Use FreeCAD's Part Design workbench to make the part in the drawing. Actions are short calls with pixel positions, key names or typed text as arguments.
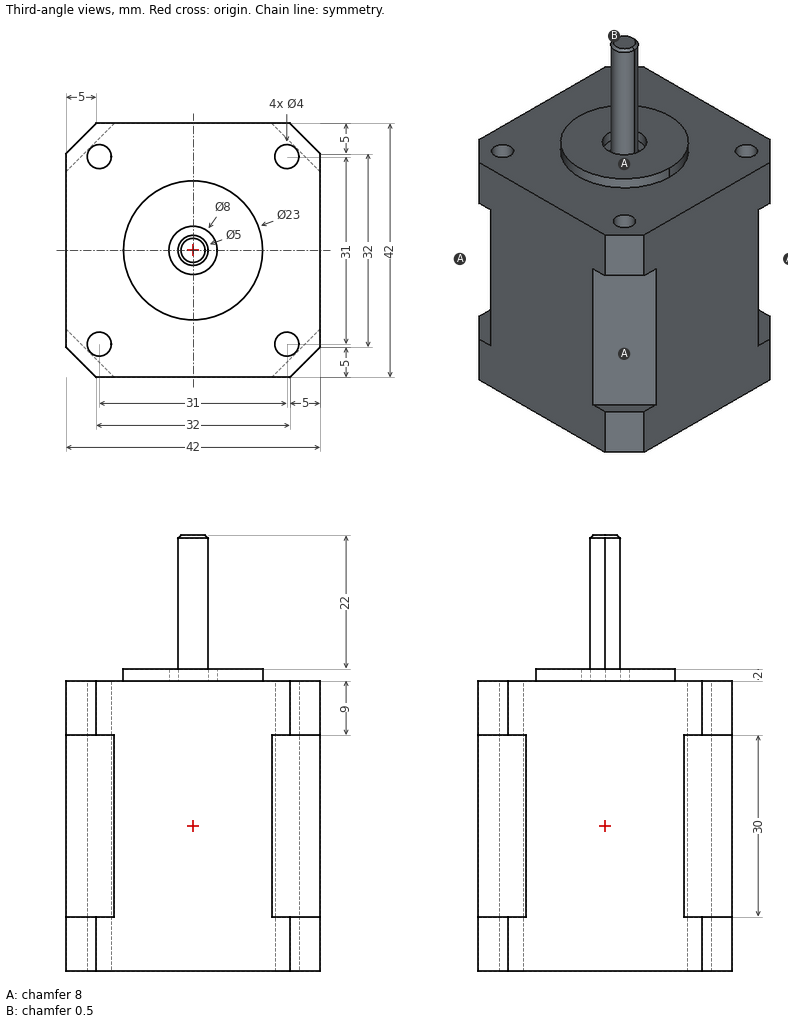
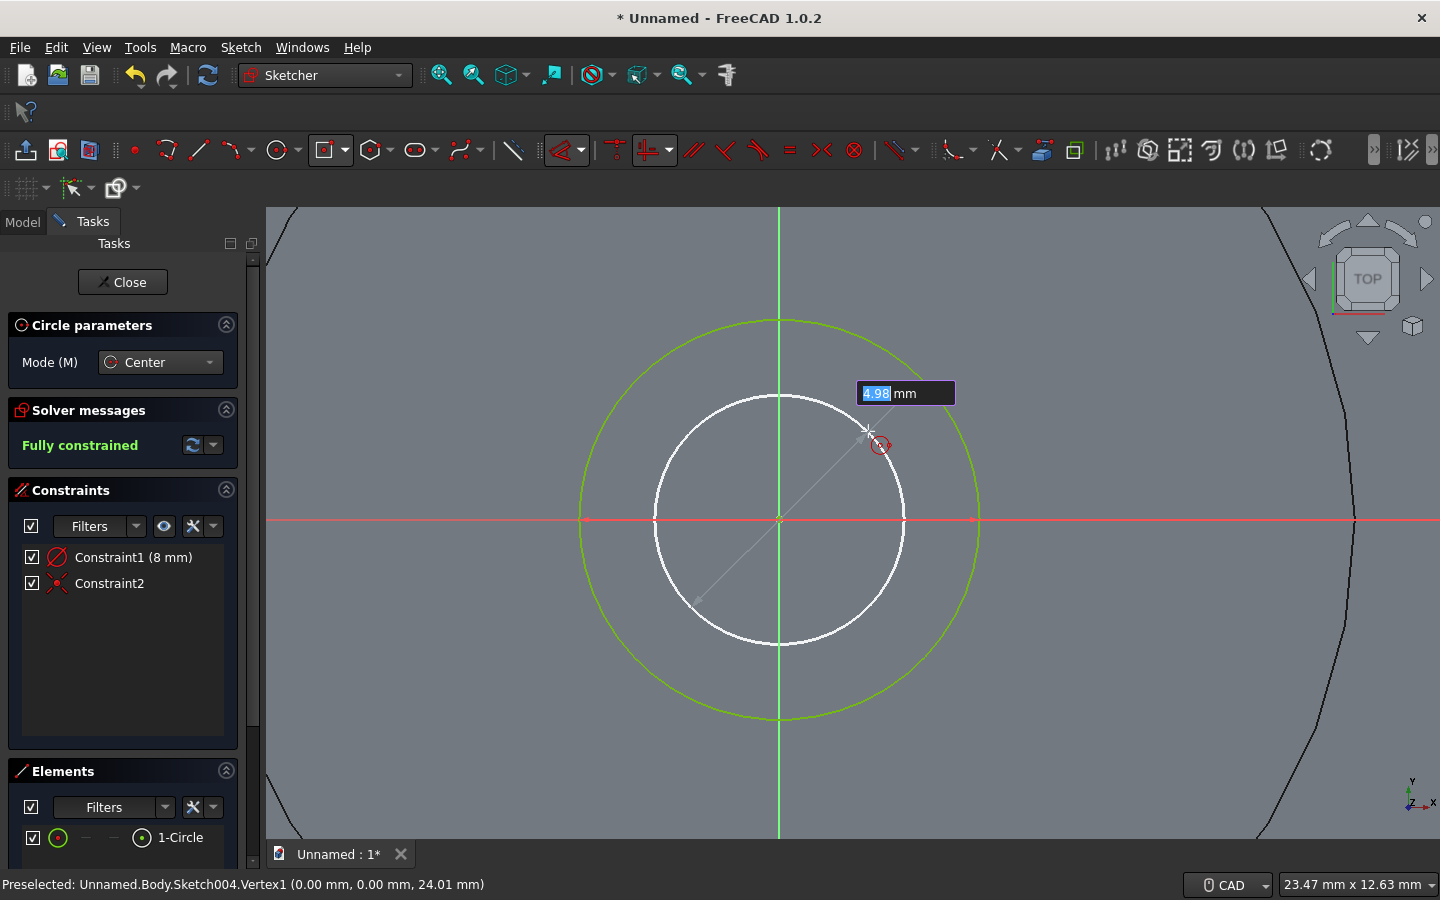
text(5)
key(Return)
key(Escape)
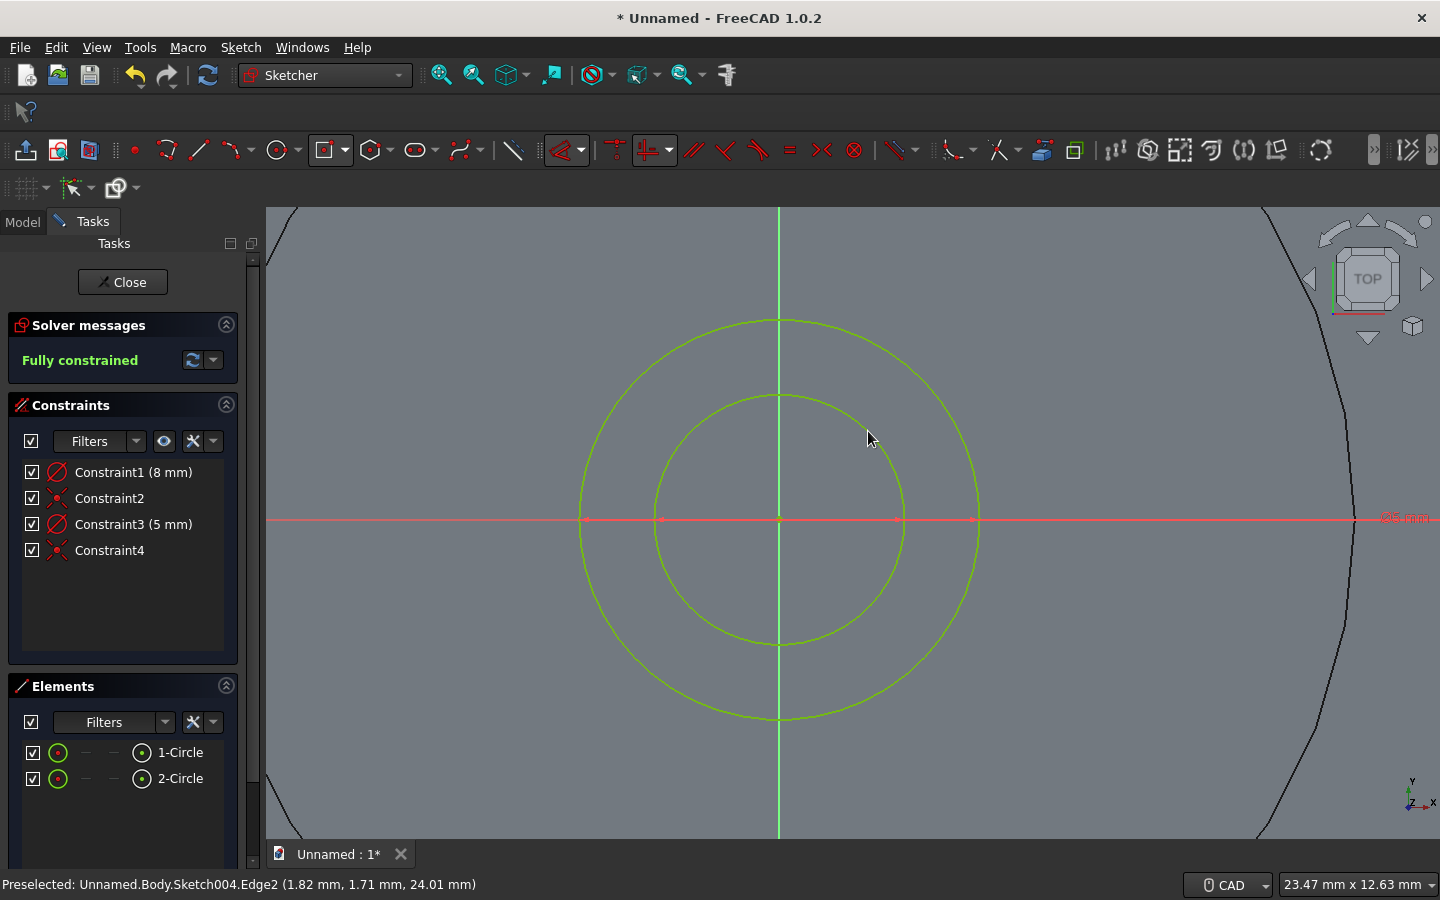
click(123, 282)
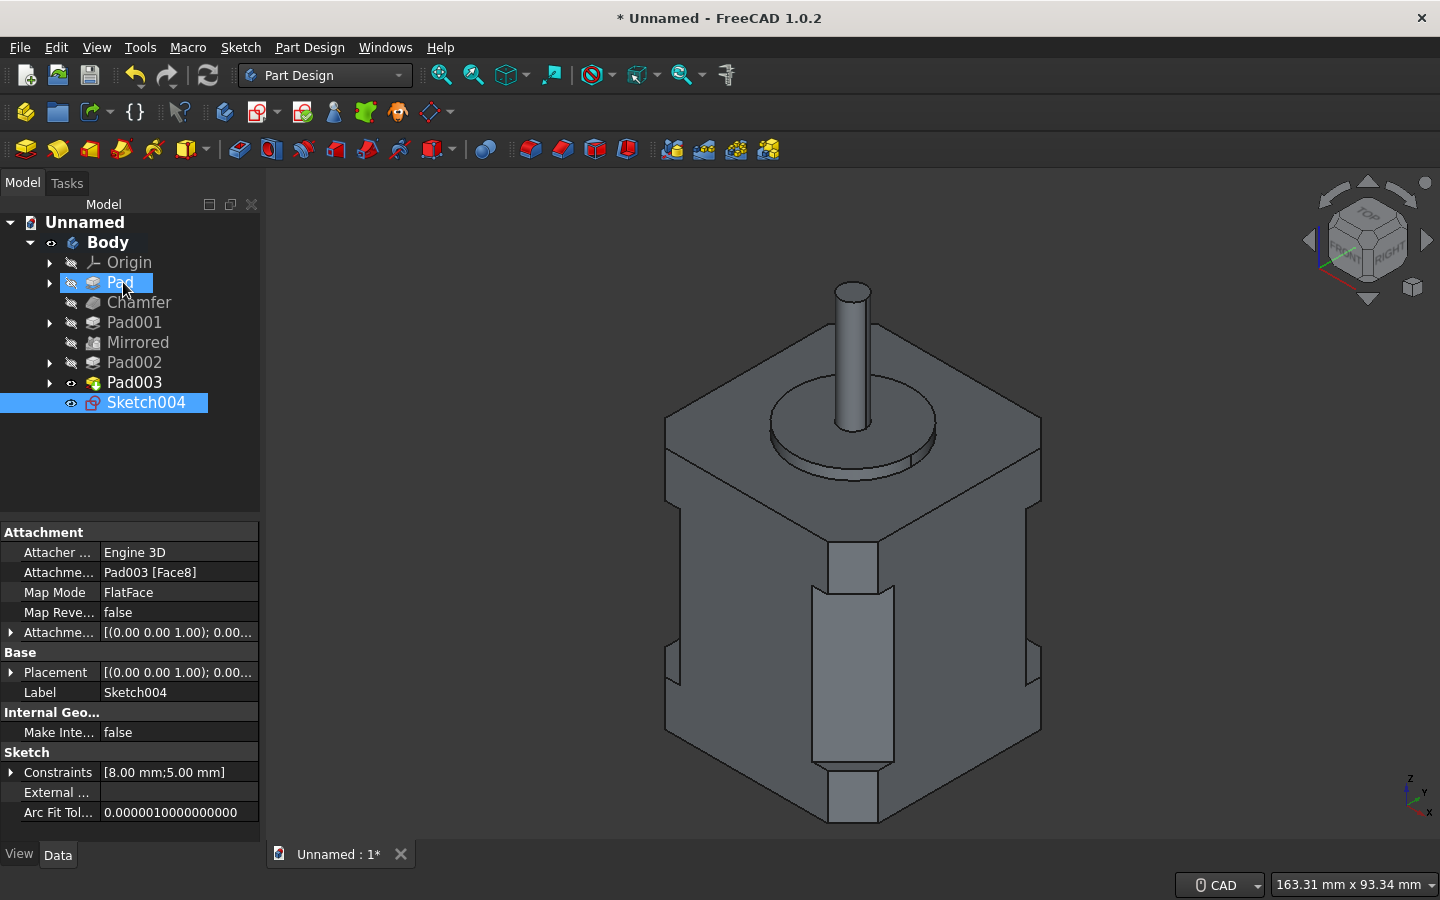
click(240, 150)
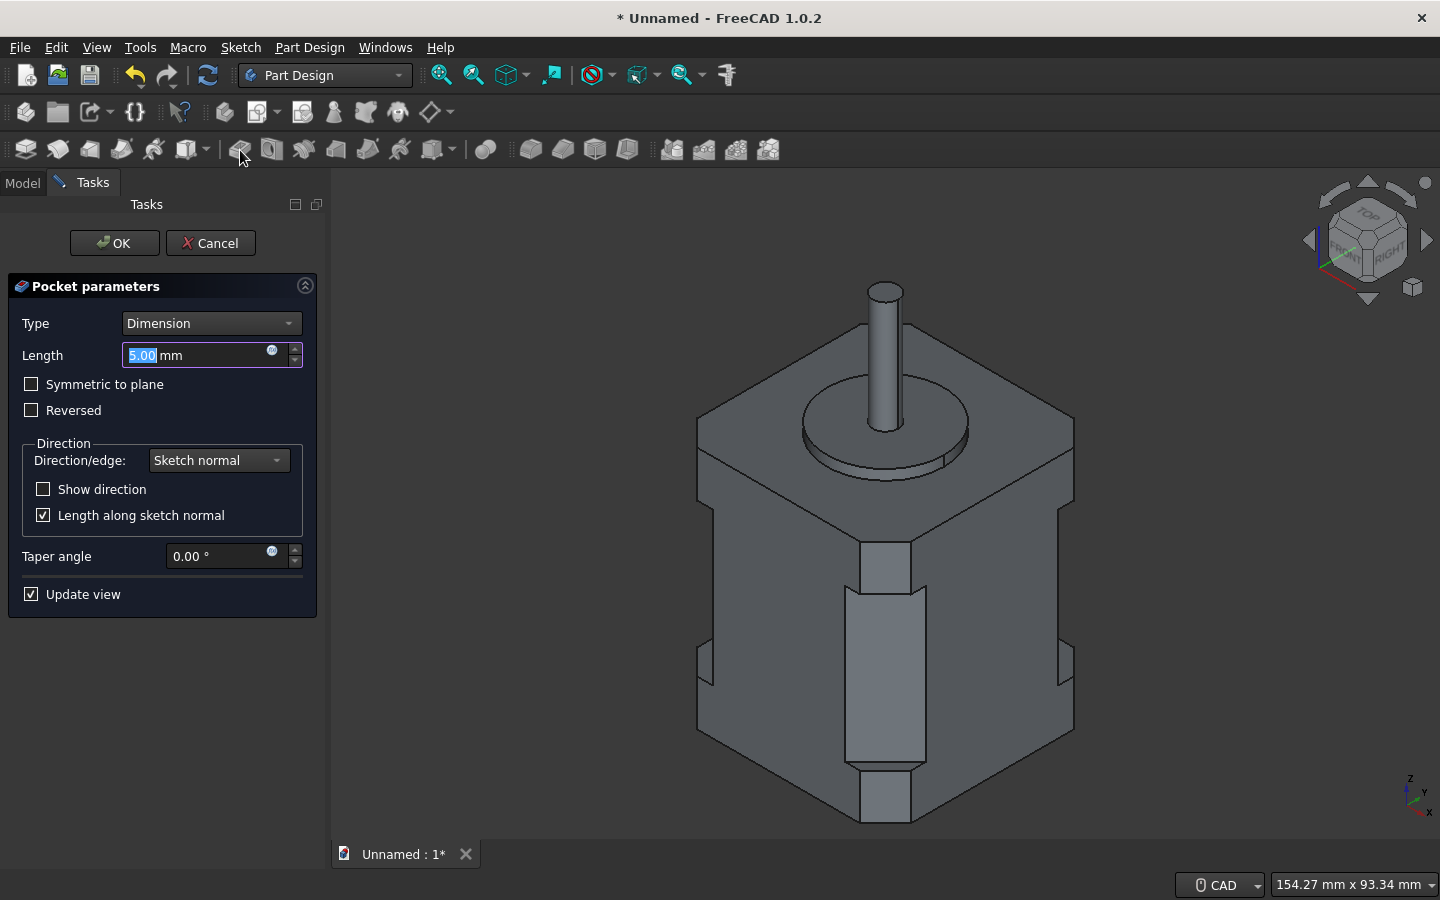
text(2)
key(Tab)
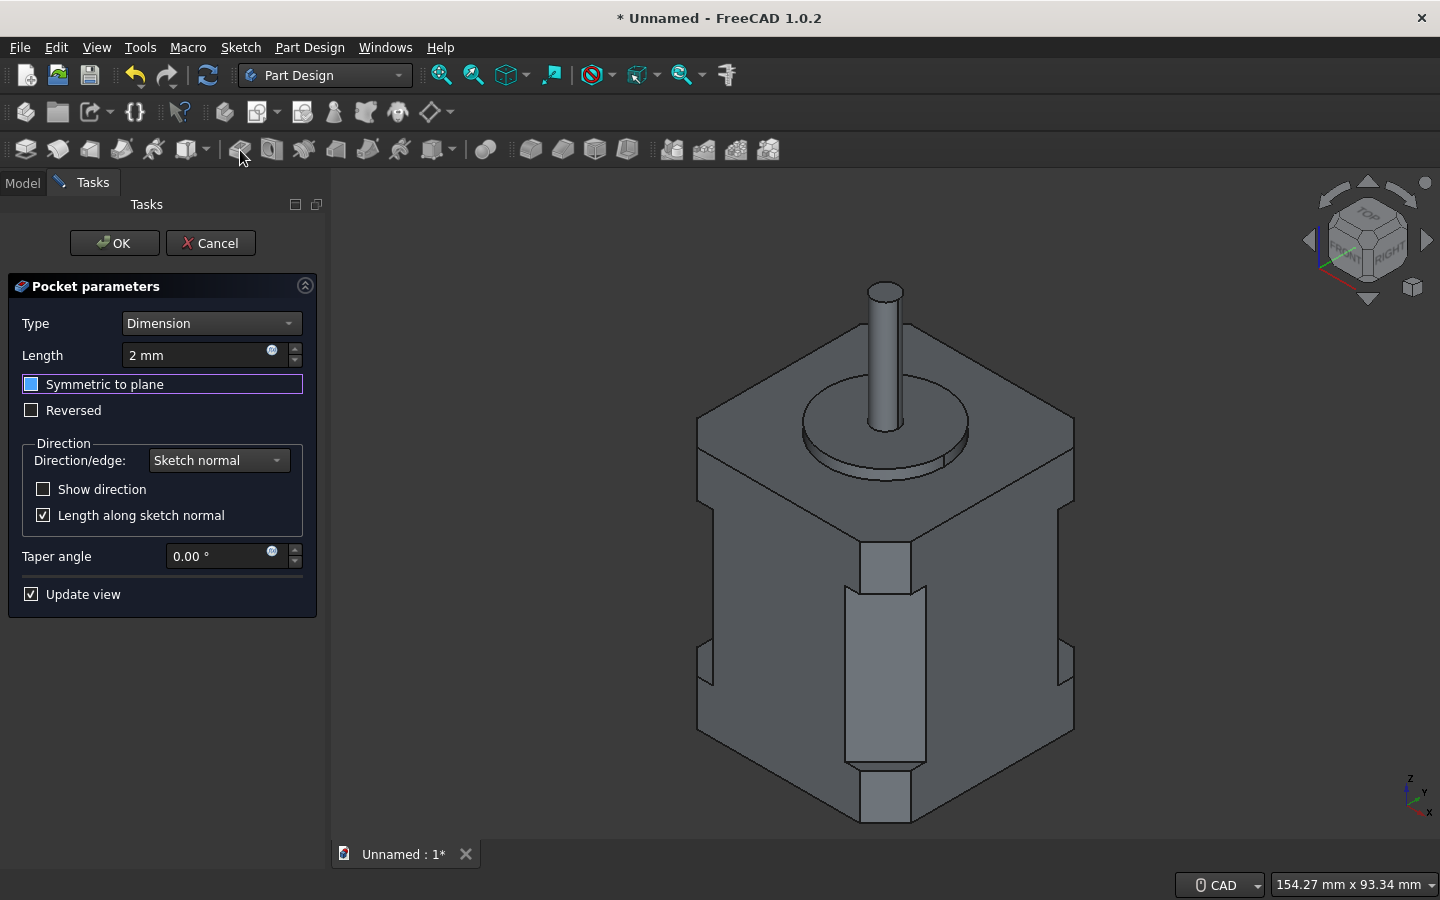
click(30, 410)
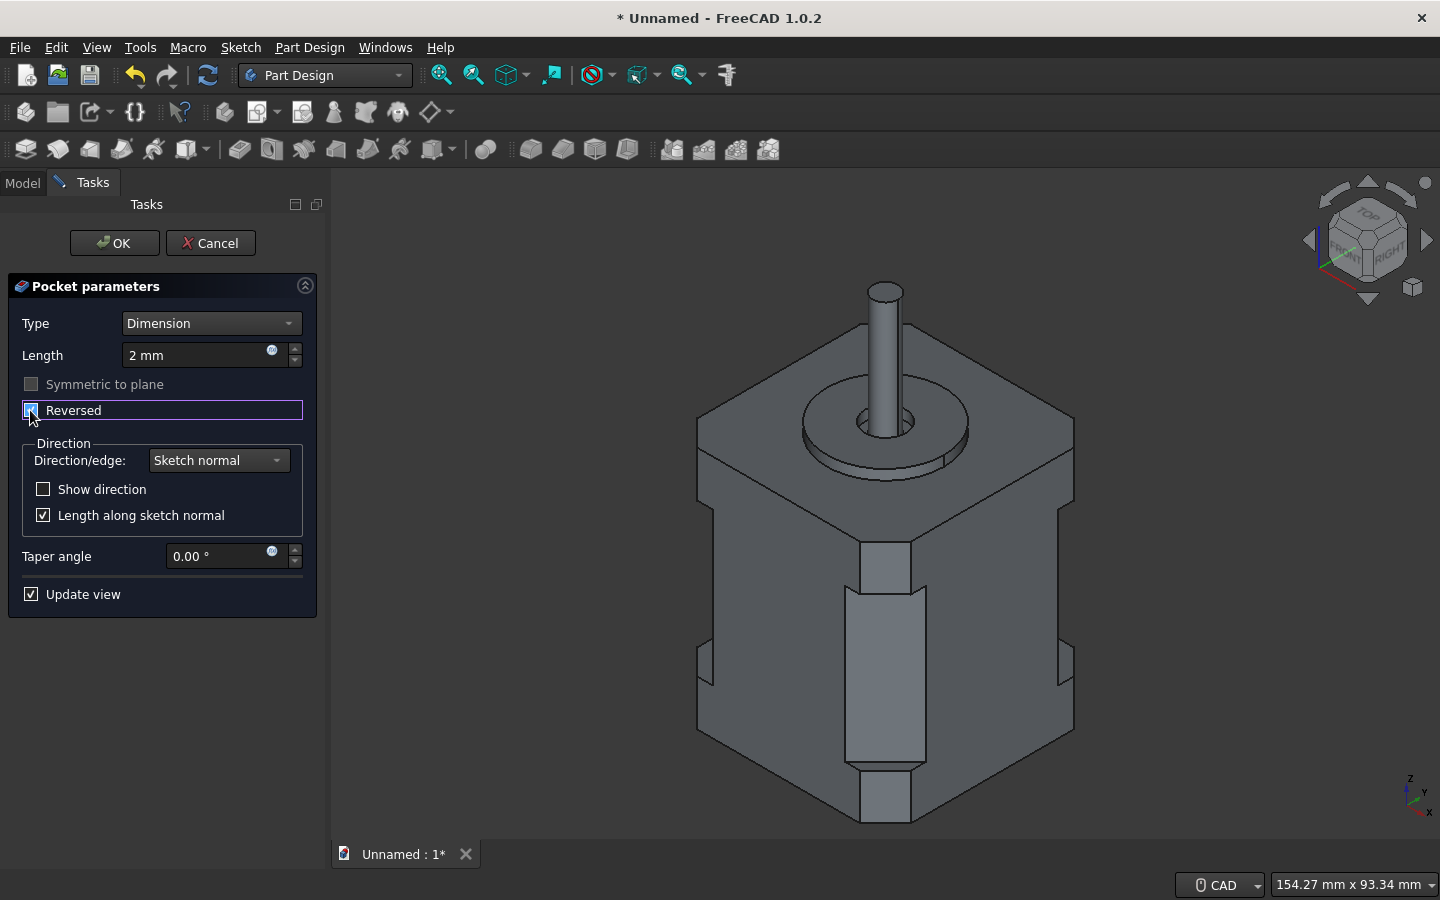
click(115, 243)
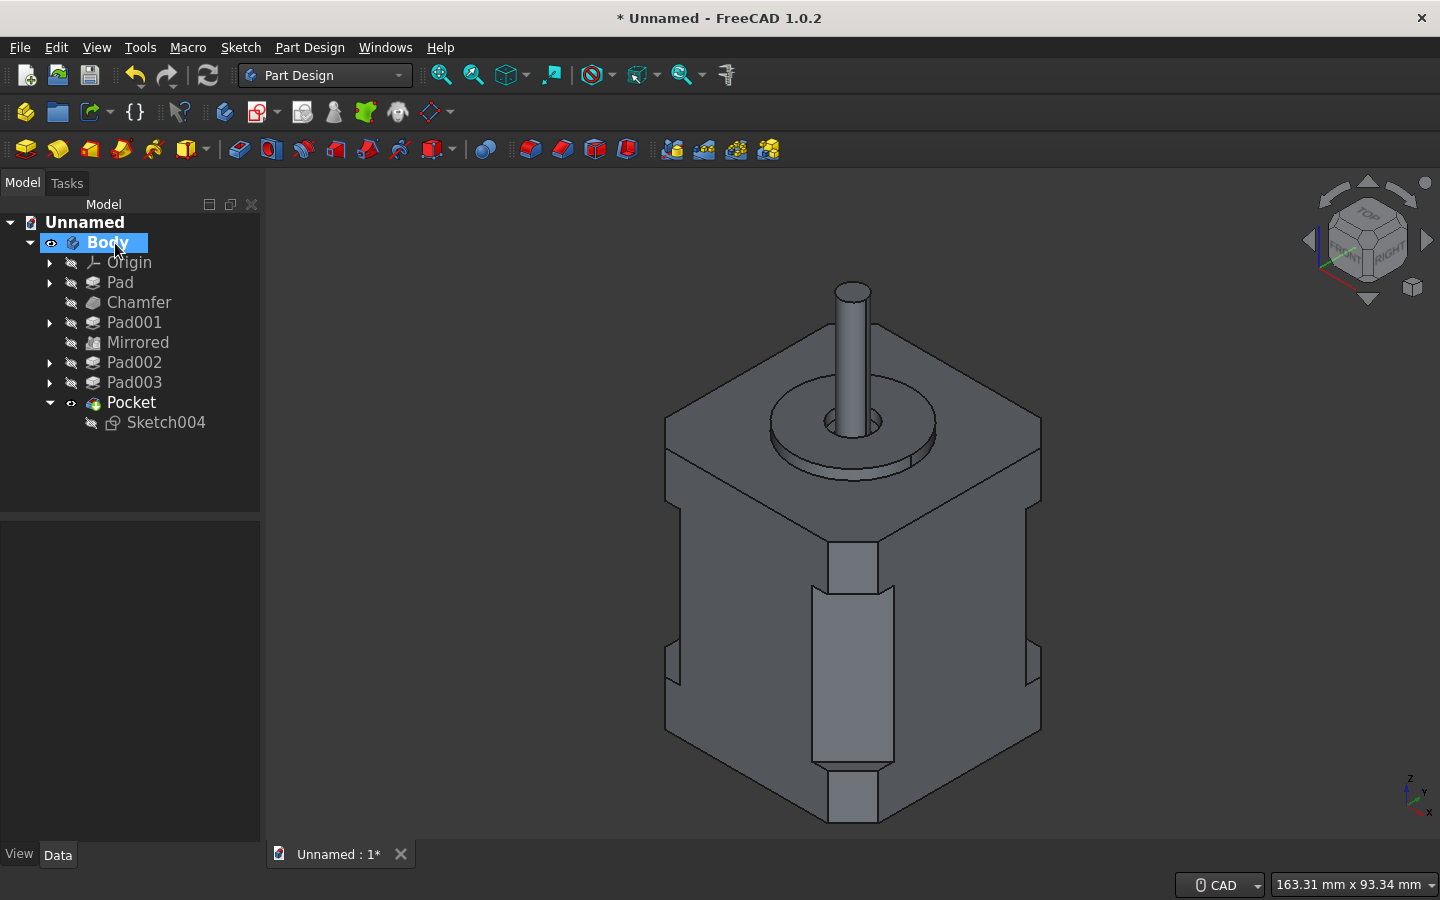
click(840, 284)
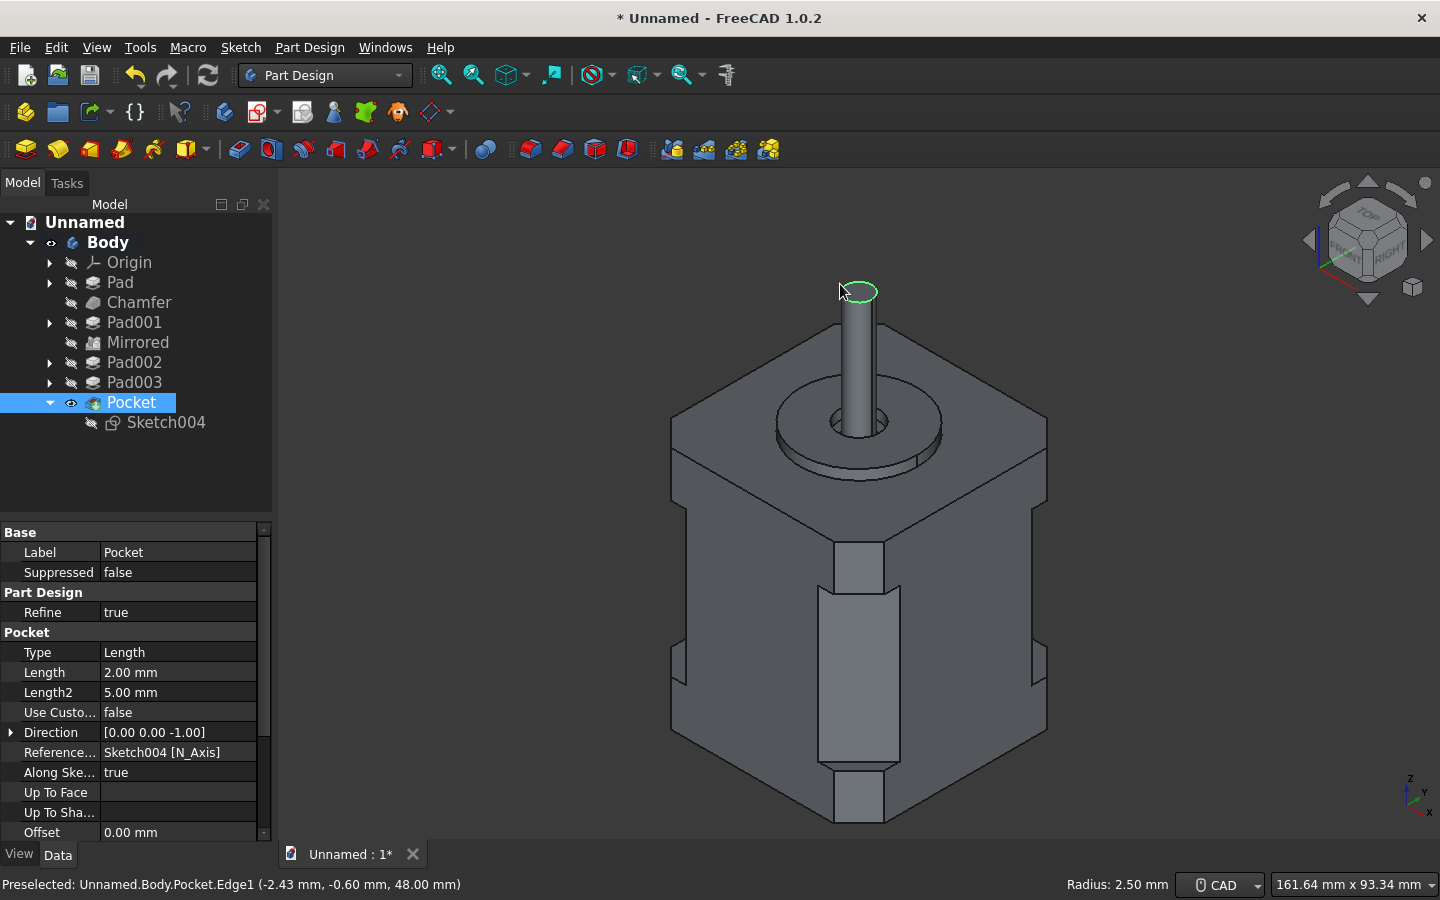
click(564, 150)